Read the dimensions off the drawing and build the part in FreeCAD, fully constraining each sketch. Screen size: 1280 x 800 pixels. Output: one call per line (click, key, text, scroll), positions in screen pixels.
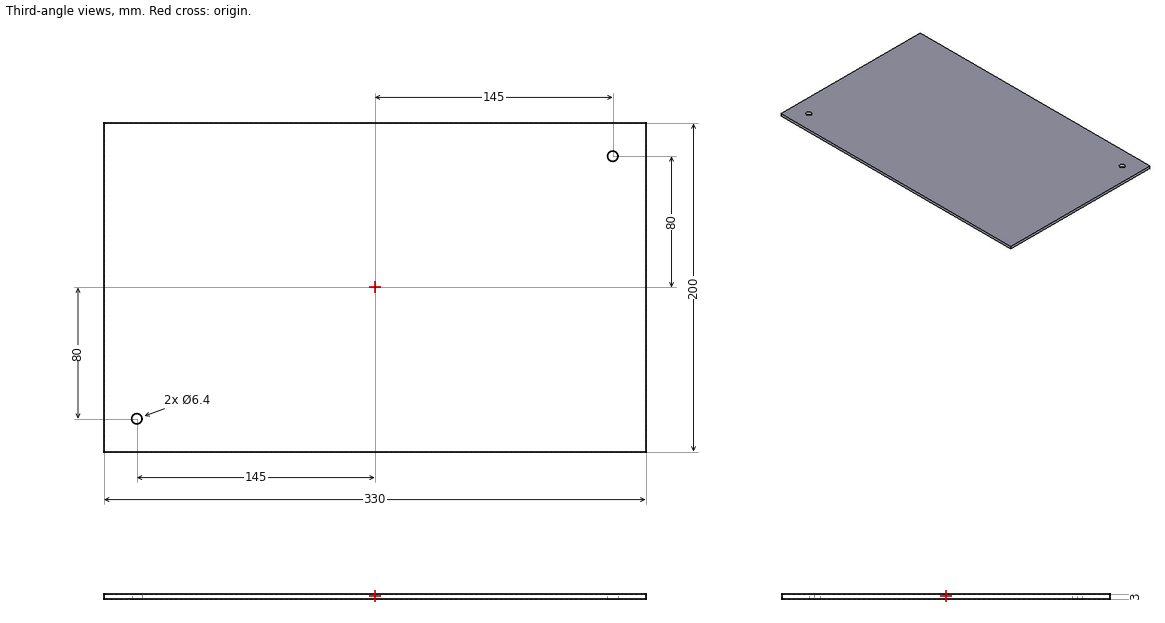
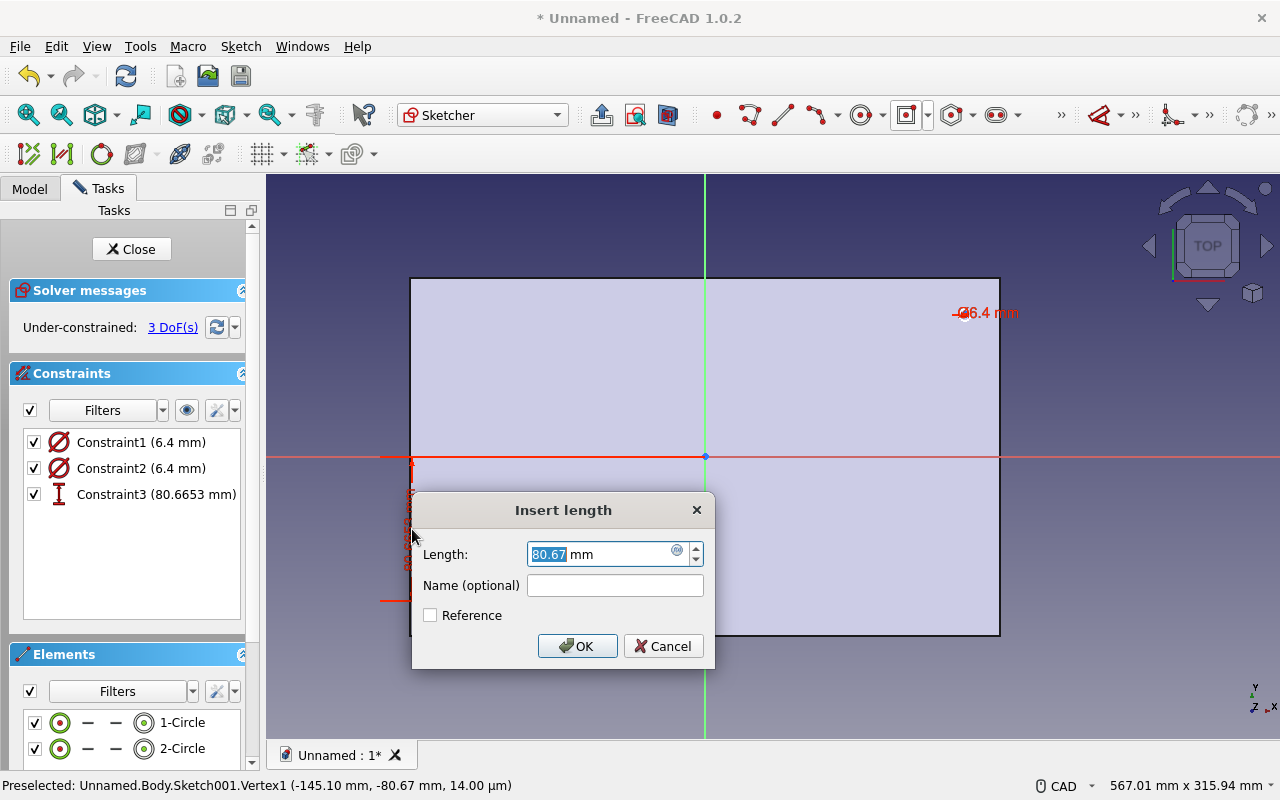
text(80)
key(Return)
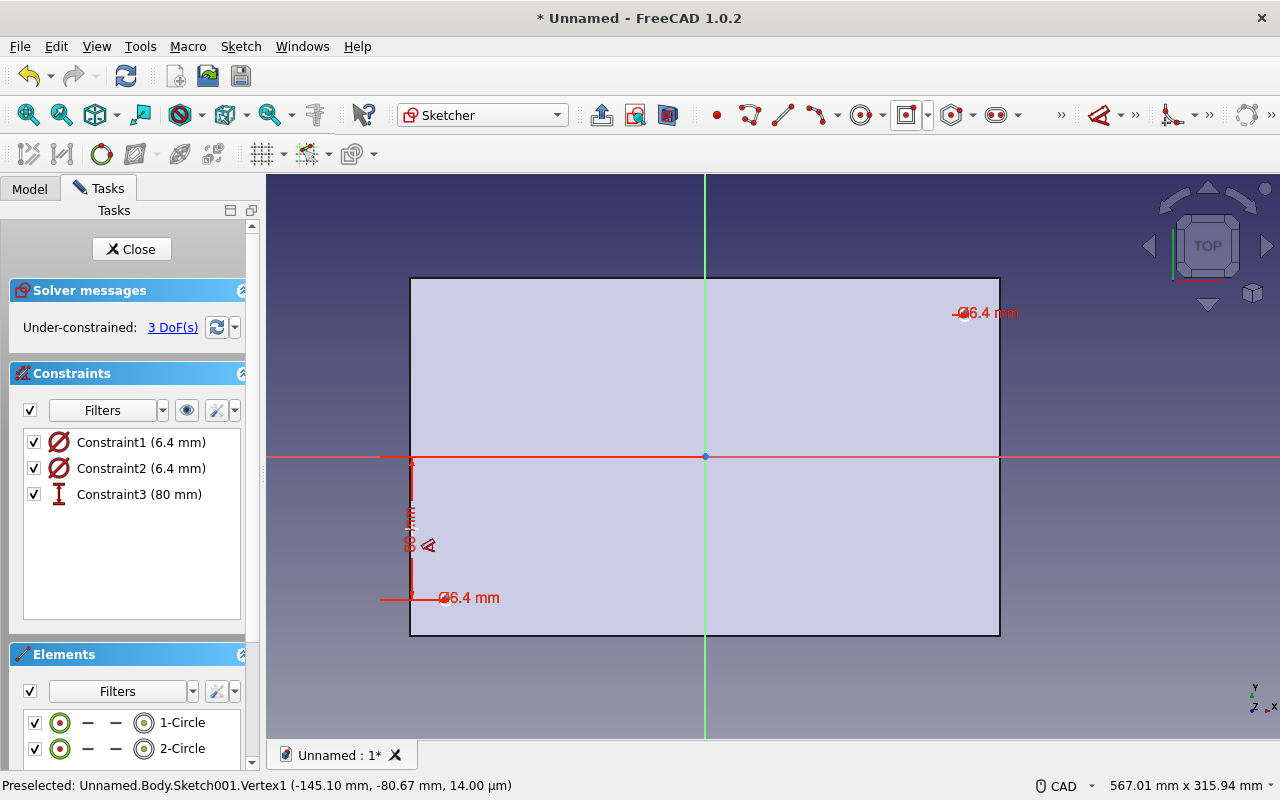
click(965, 315)
click(999, 386)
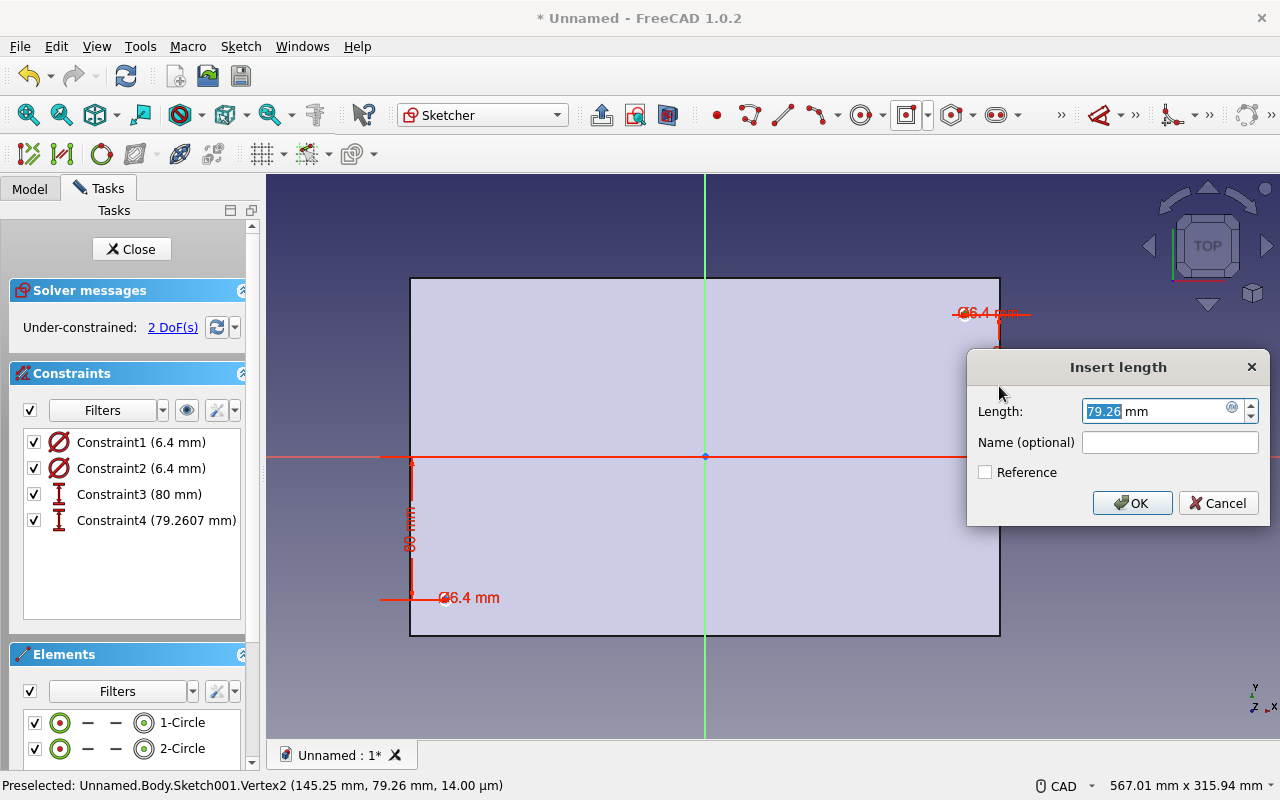
text(80)
key(Return)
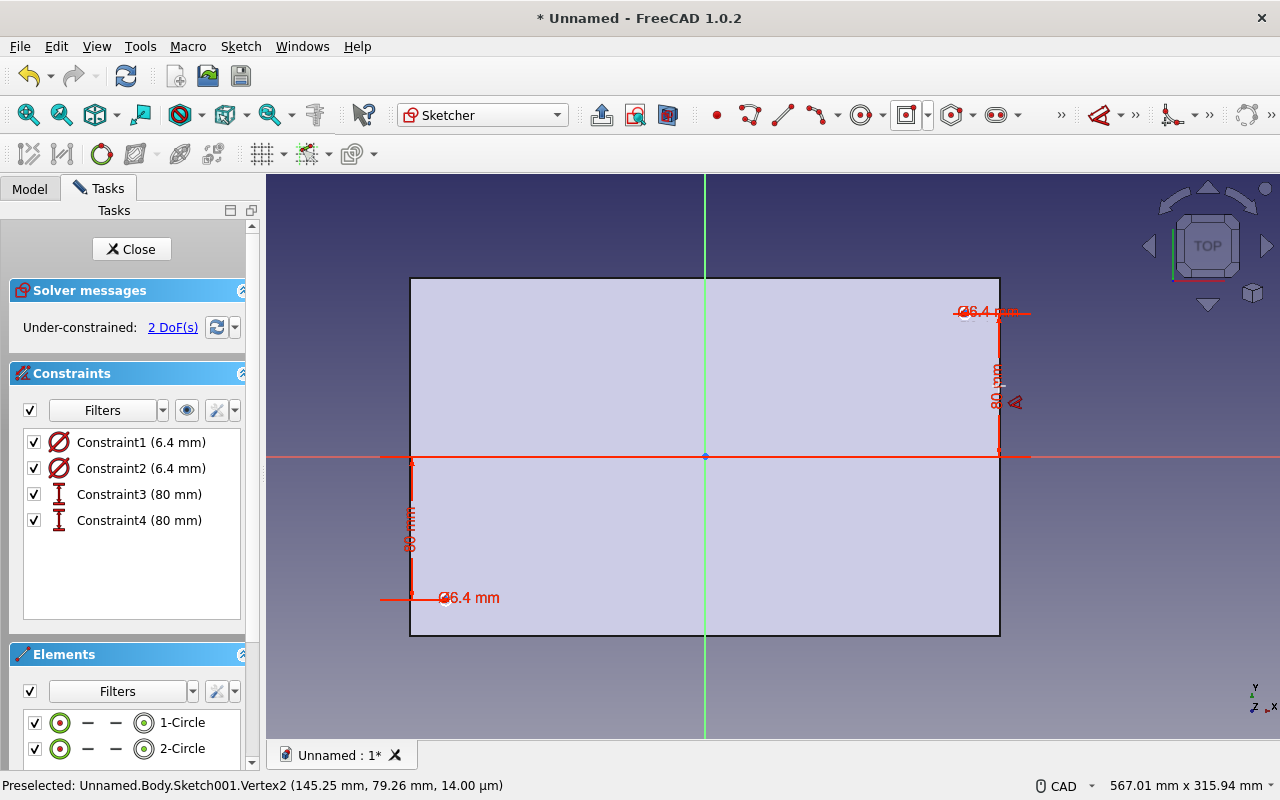
click(446, 600)
click(575, 634)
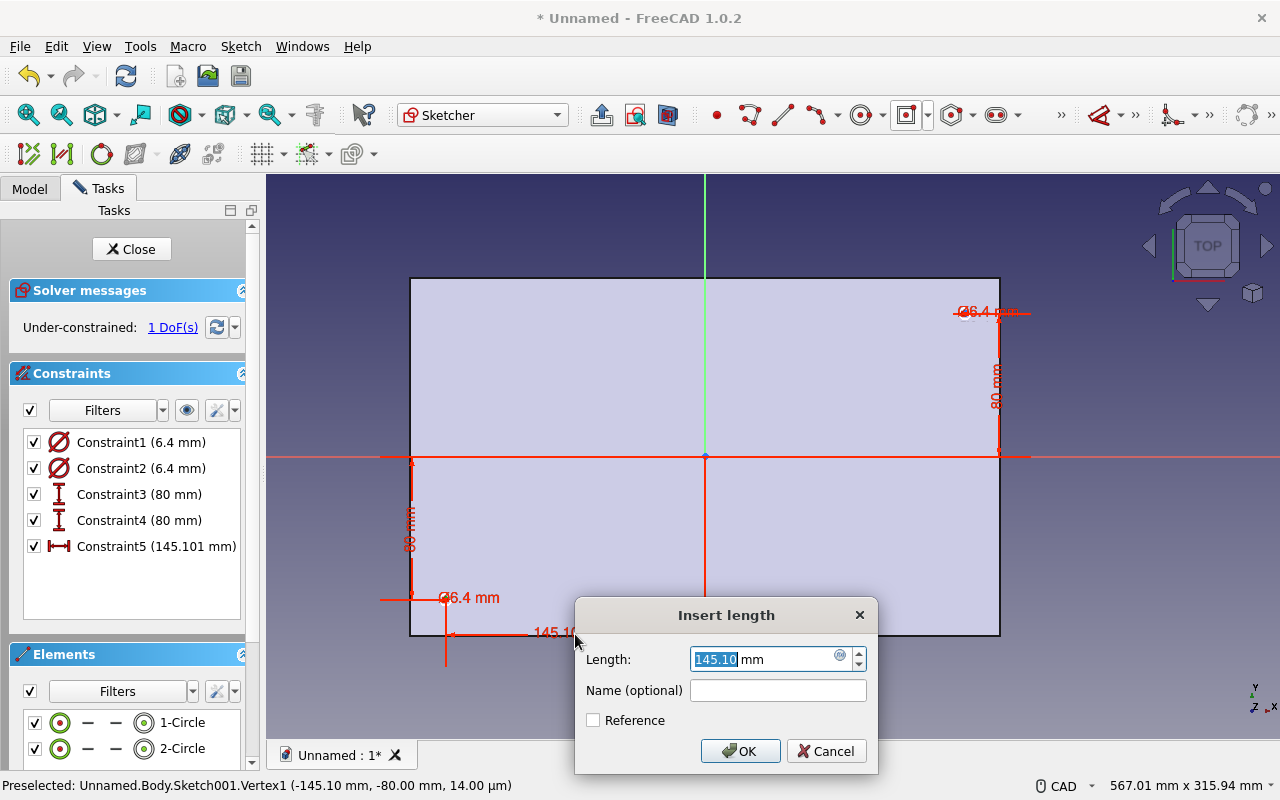
text(145)
key(Return)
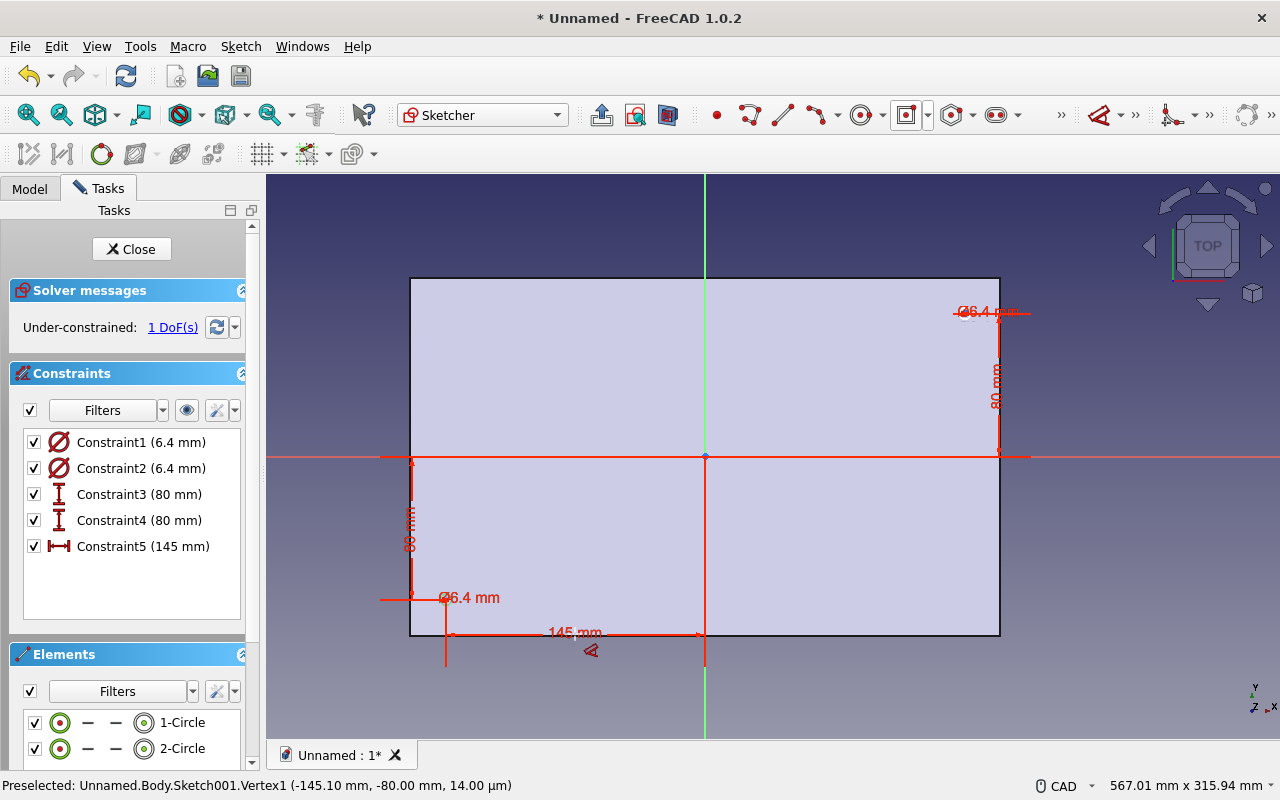
click(965, 314)
click(835, 280)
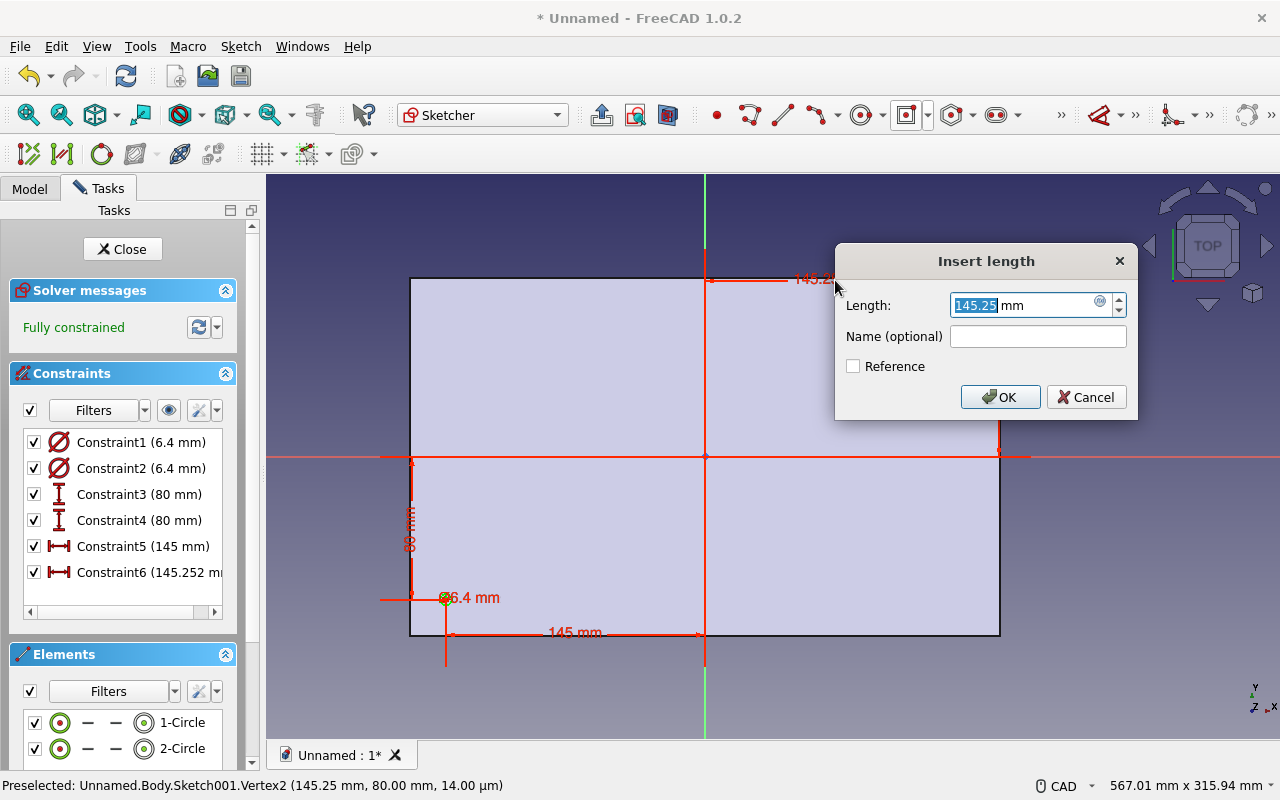
text(145)
key(Return)
key(Escape)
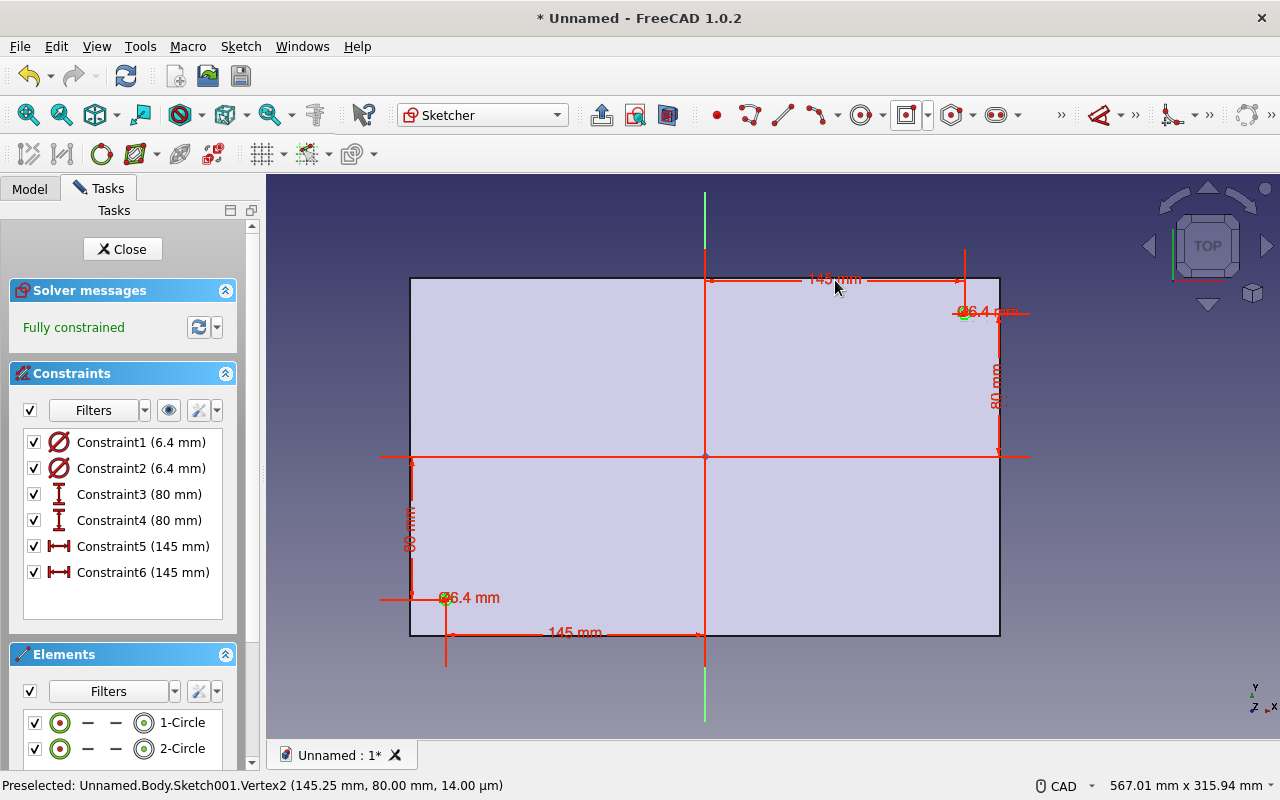
click(123, 249)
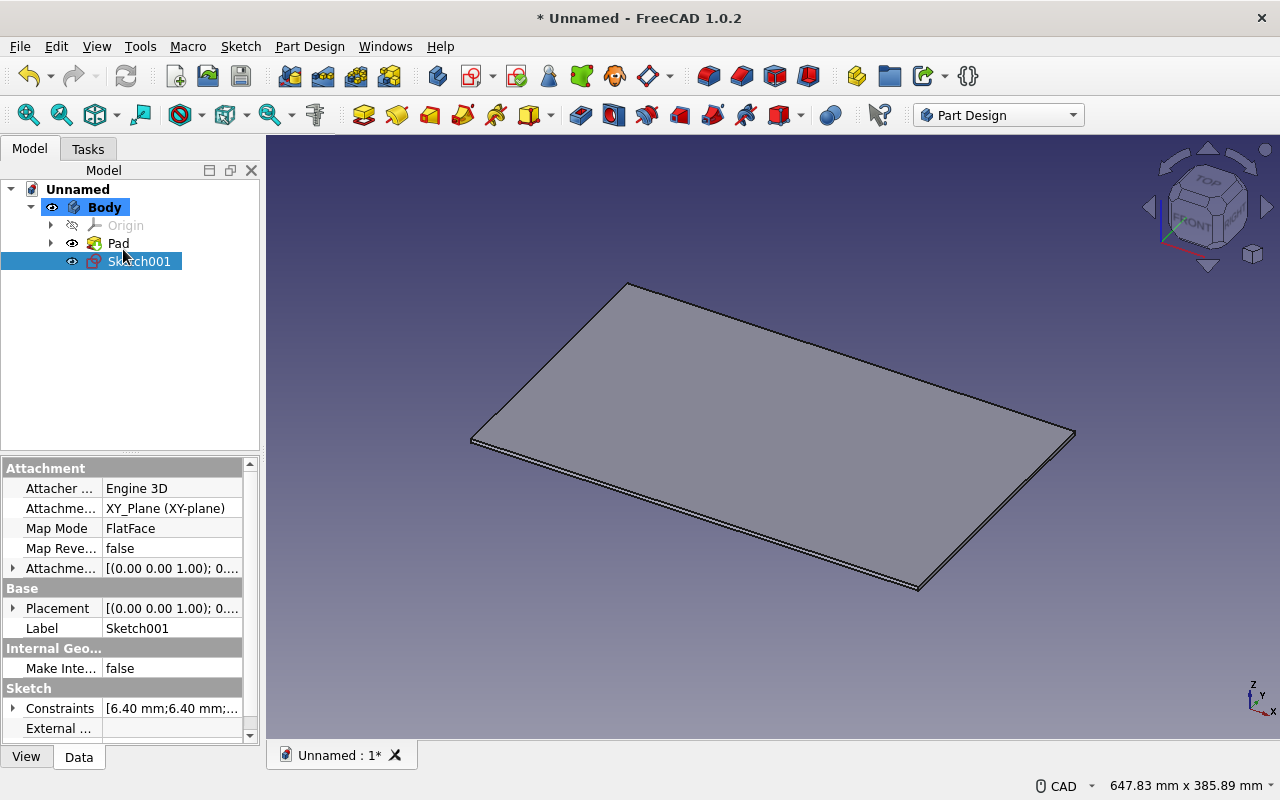
click(581, 116)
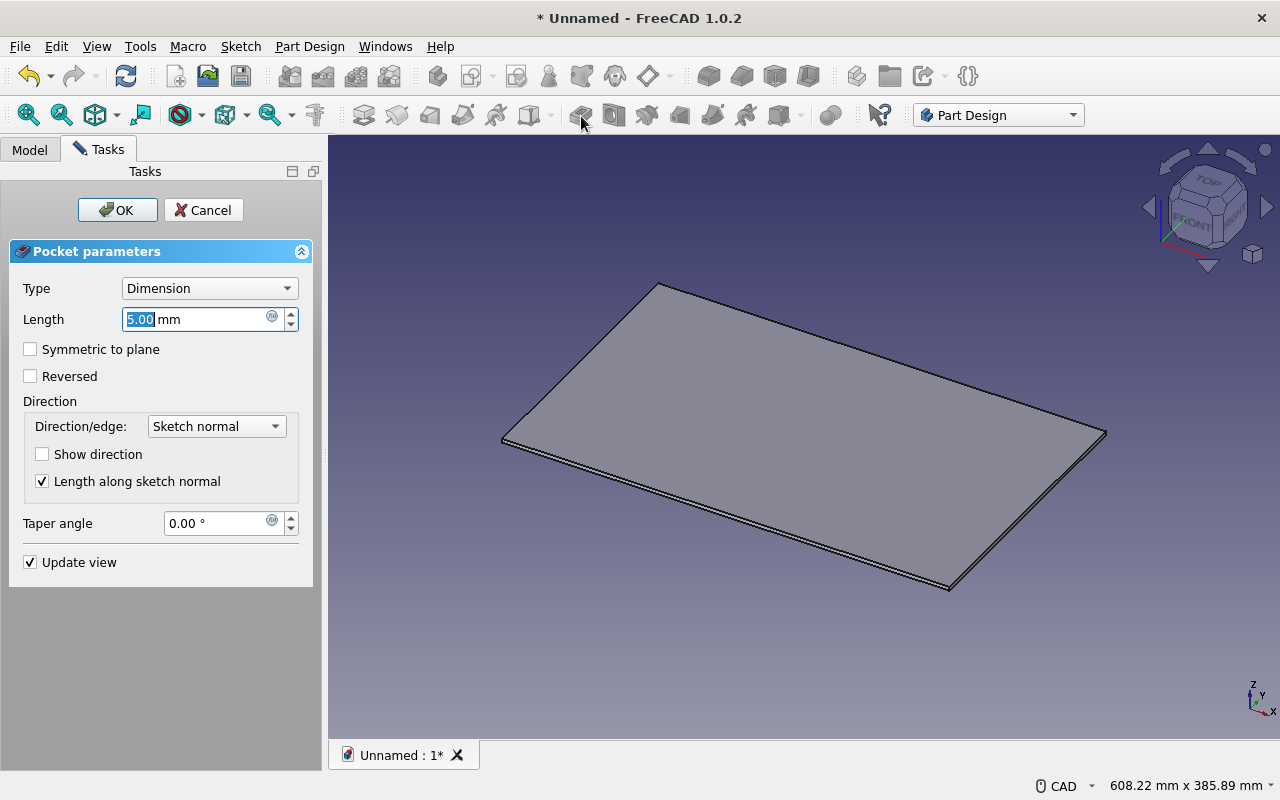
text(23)
key(Tab)